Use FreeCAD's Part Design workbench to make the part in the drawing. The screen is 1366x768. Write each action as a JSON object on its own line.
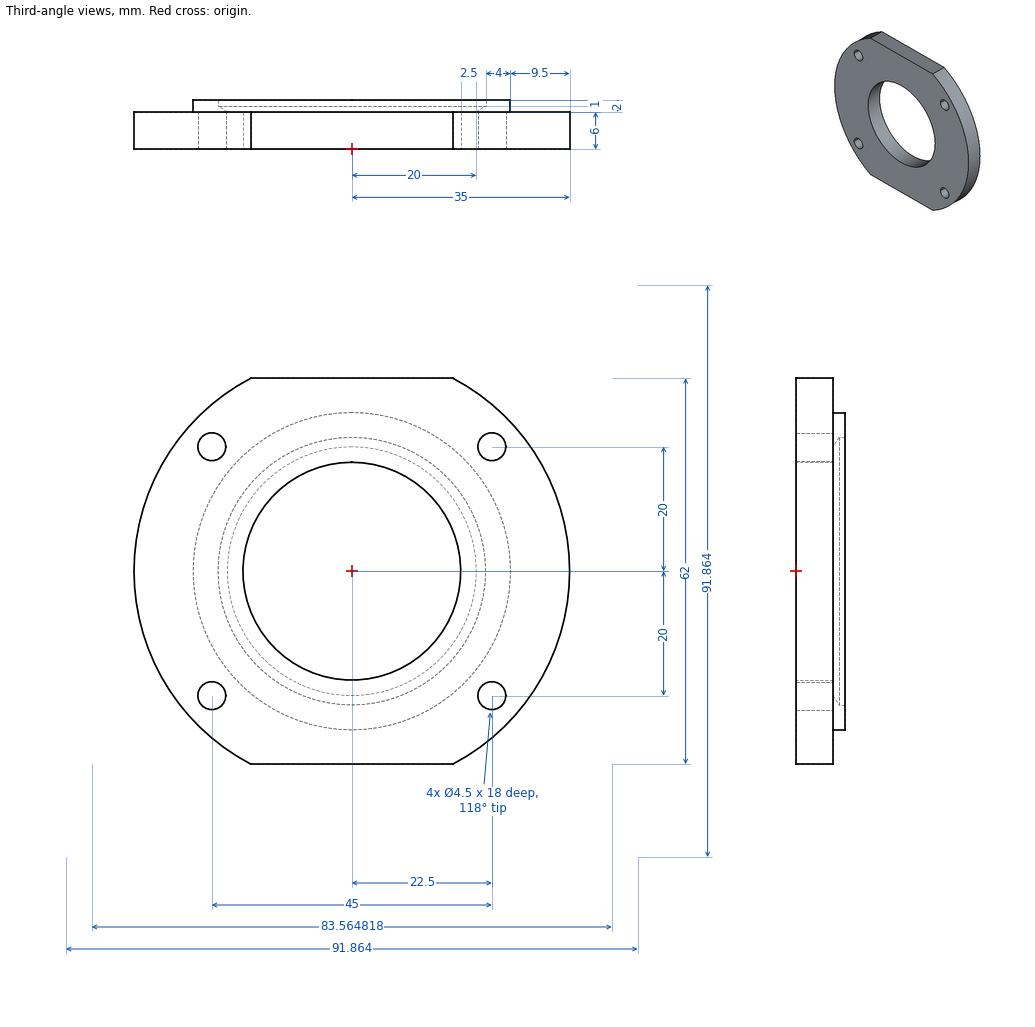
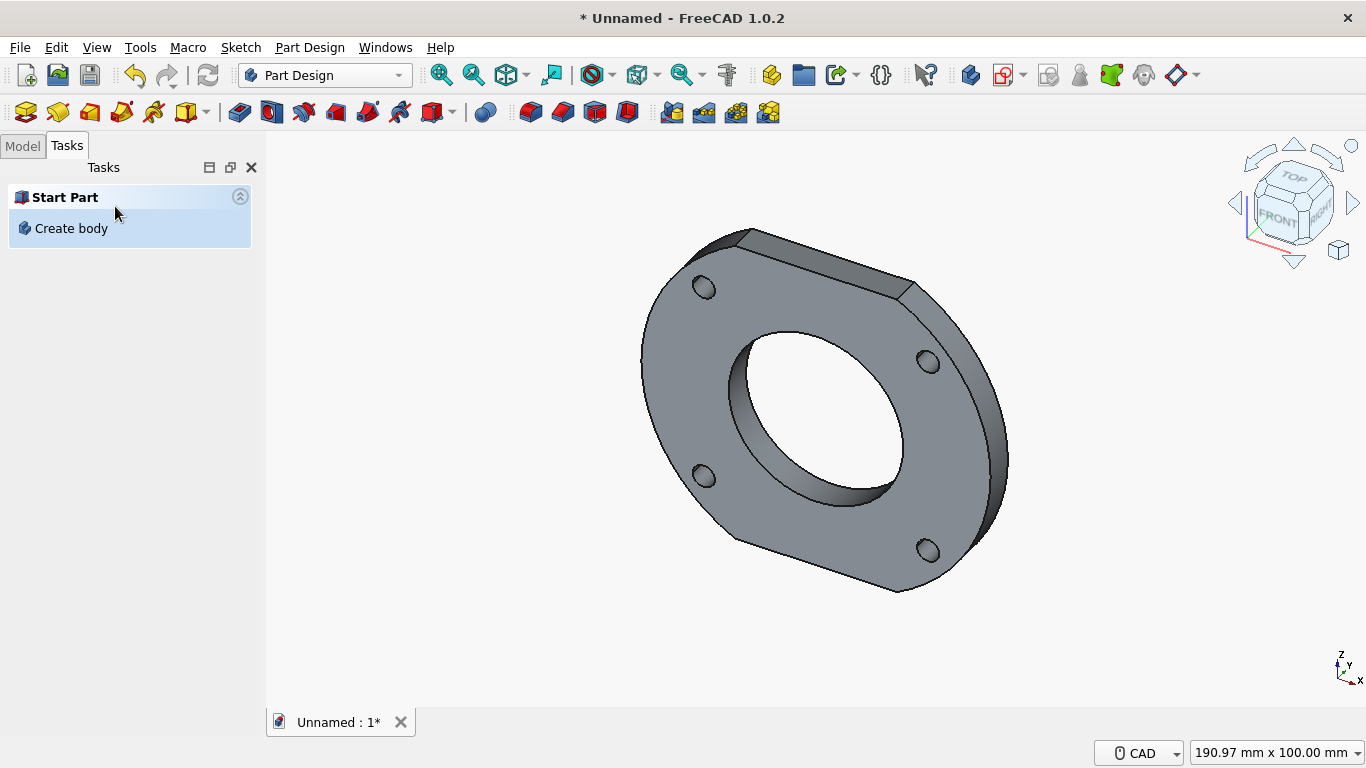
{"action": "key", "text": "0"}